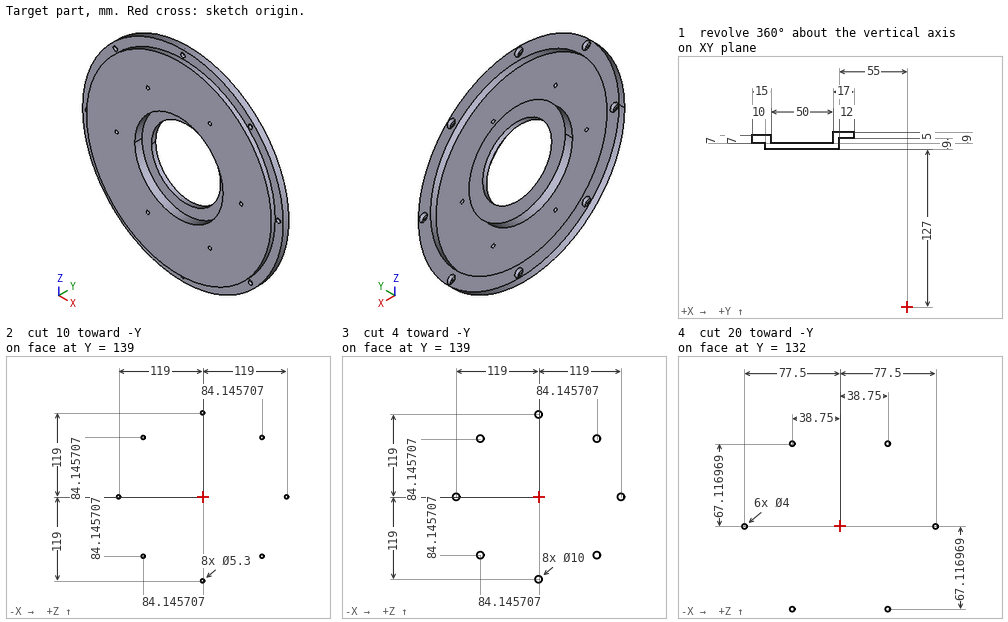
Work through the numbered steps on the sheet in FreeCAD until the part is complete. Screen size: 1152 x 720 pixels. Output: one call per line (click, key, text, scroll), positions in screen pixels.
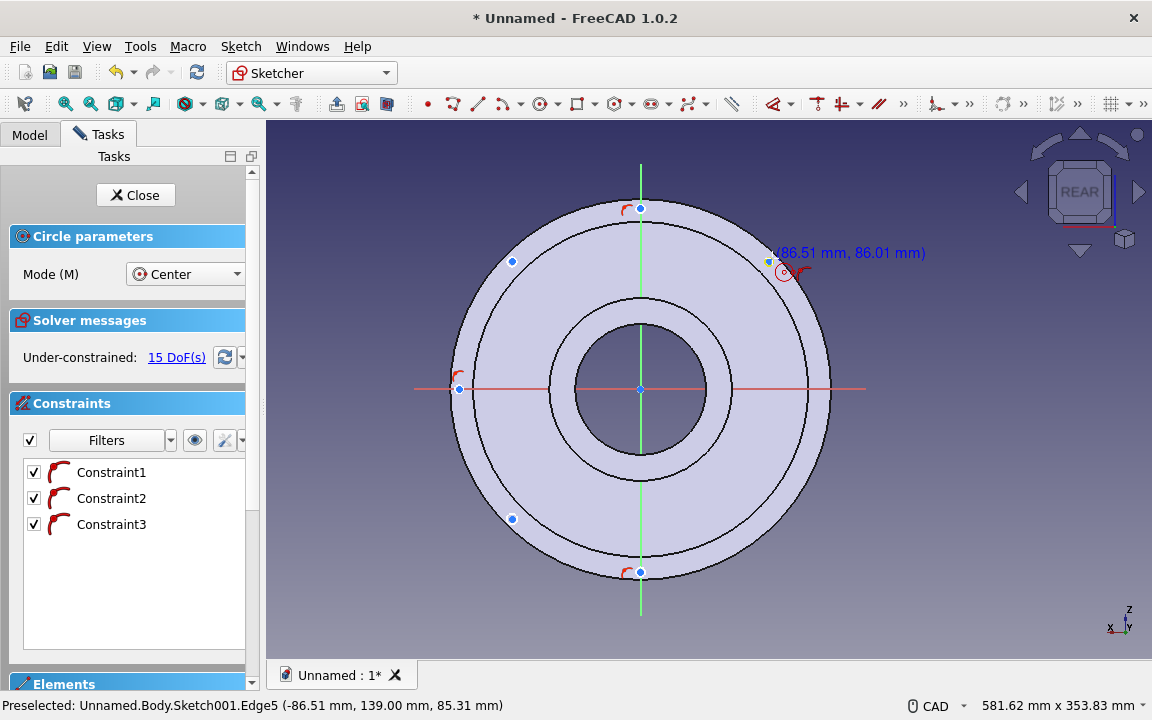
scroll(822, 389, up, 9)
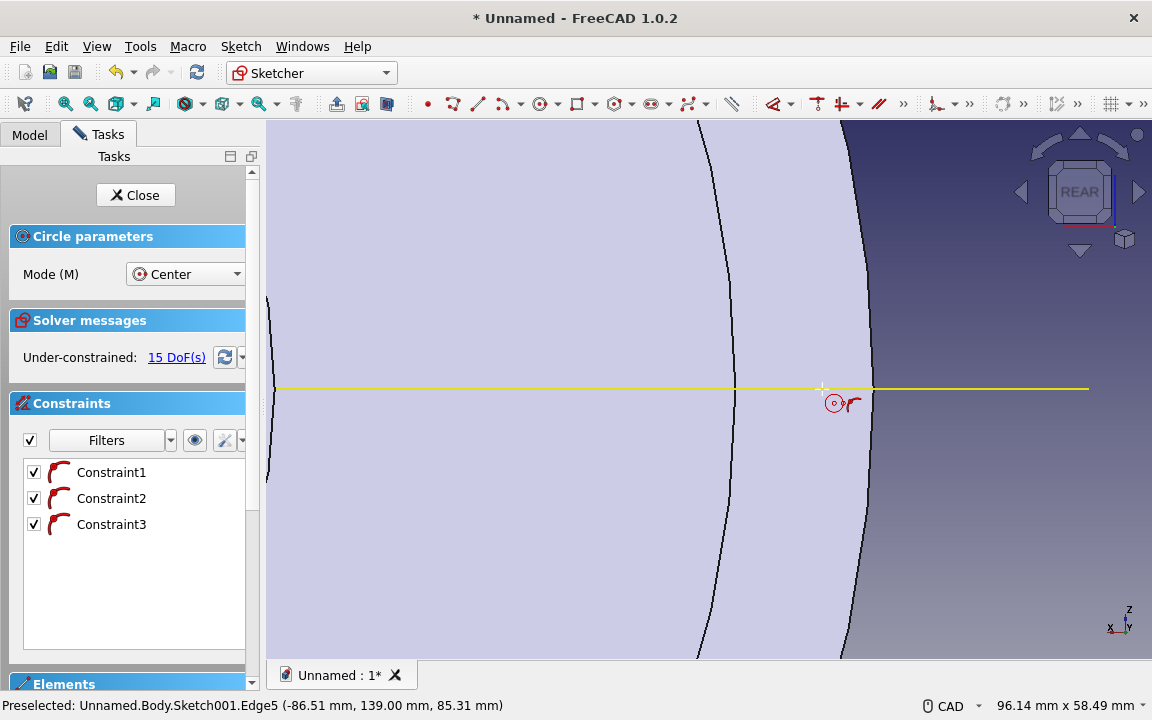
scroll(822, 390, down, 9)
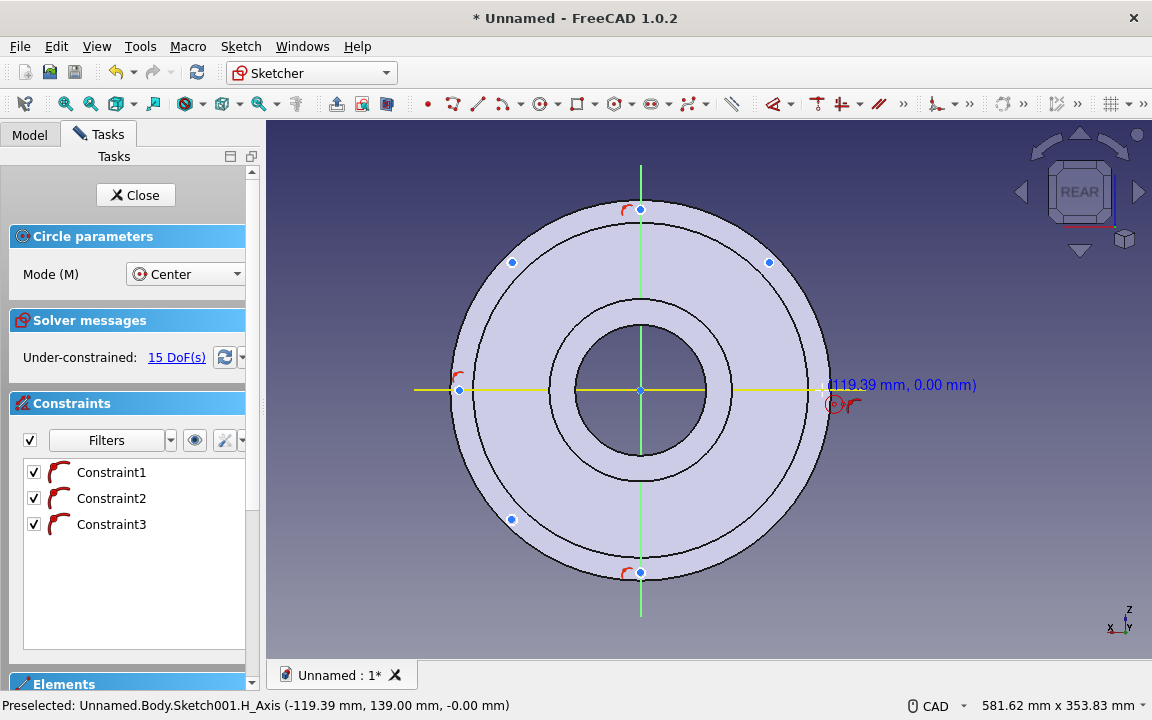
click(822, 390)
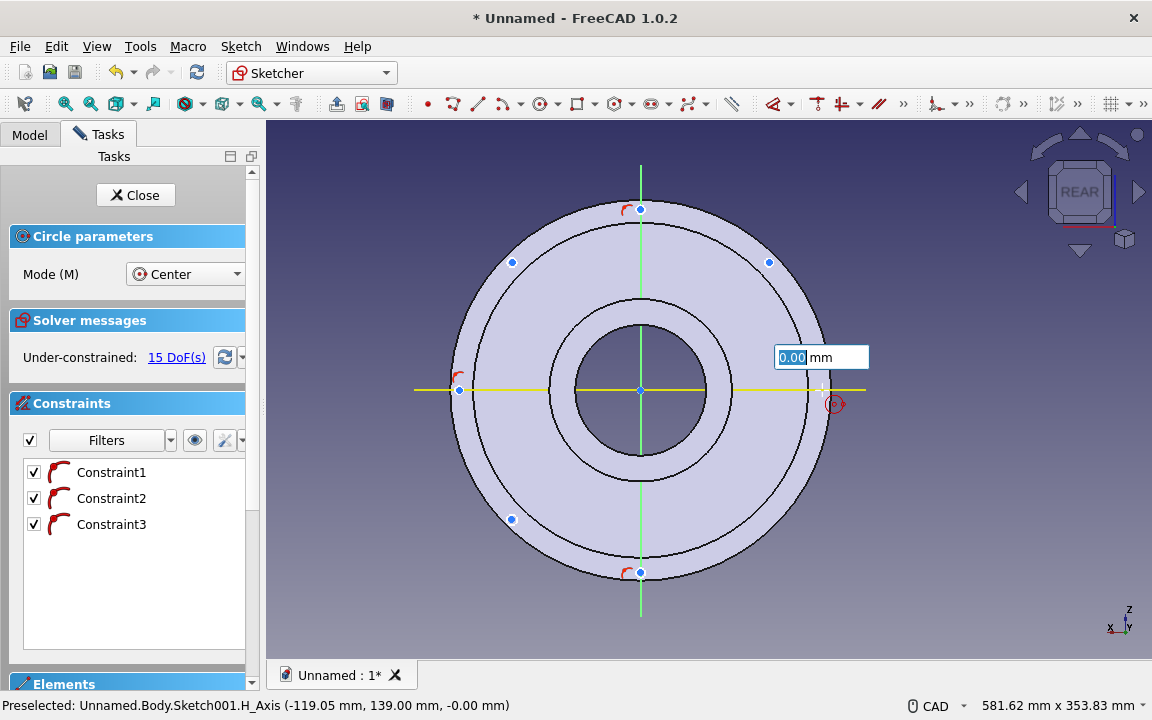
scroll(821, 394, up, 8)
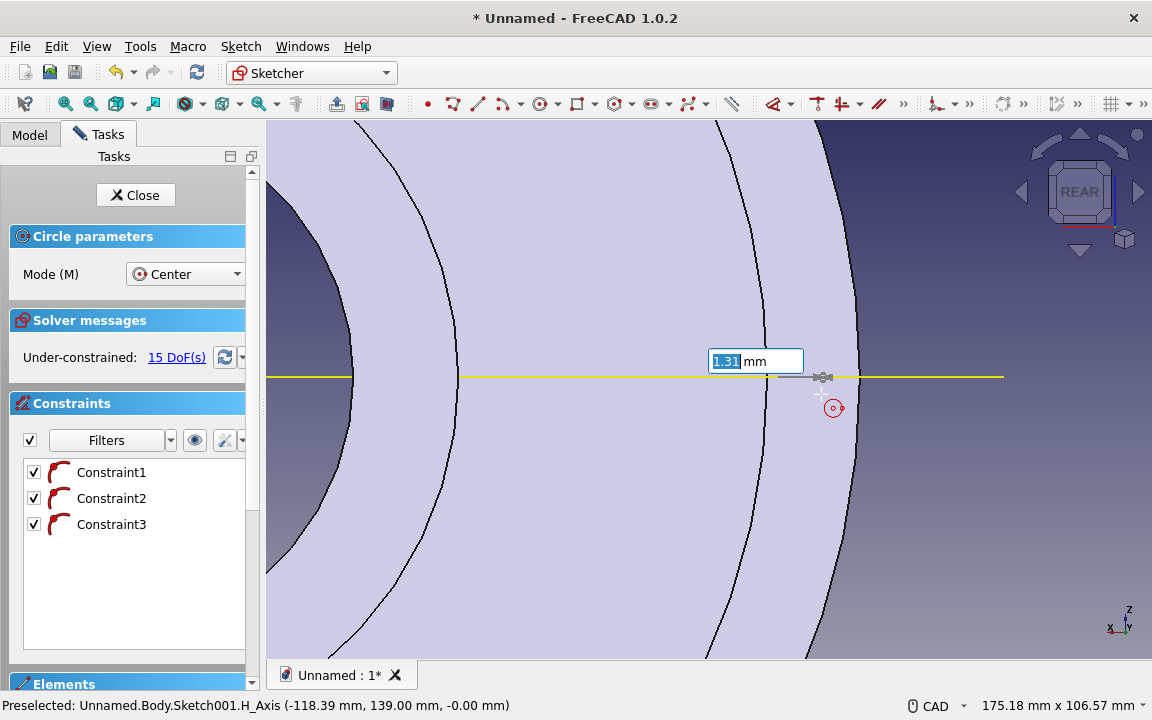
click(816, 392)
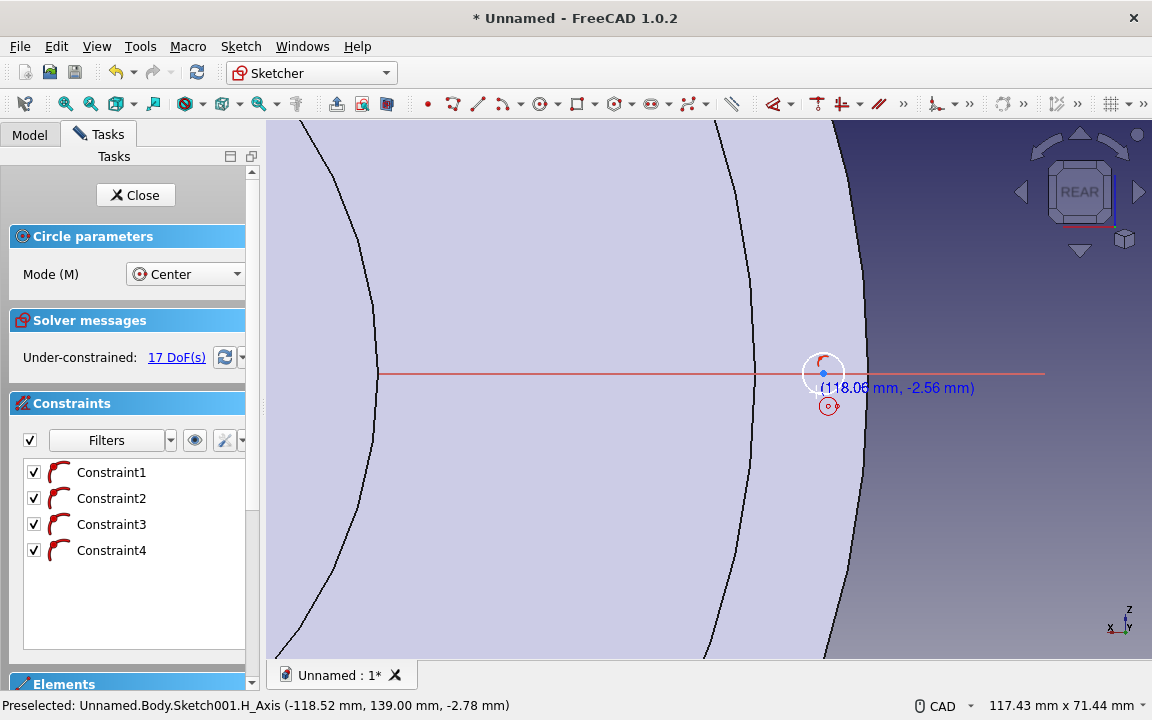
scroll(821, 394, down, 8)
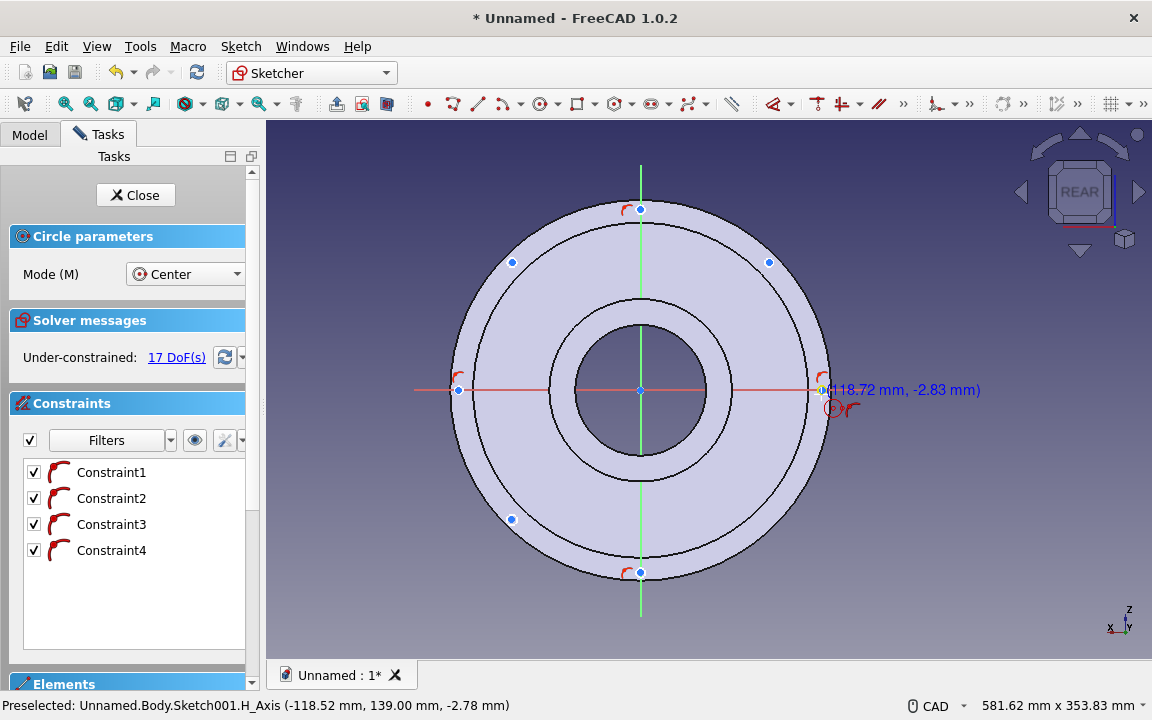
scroll(769, 518, up, 9)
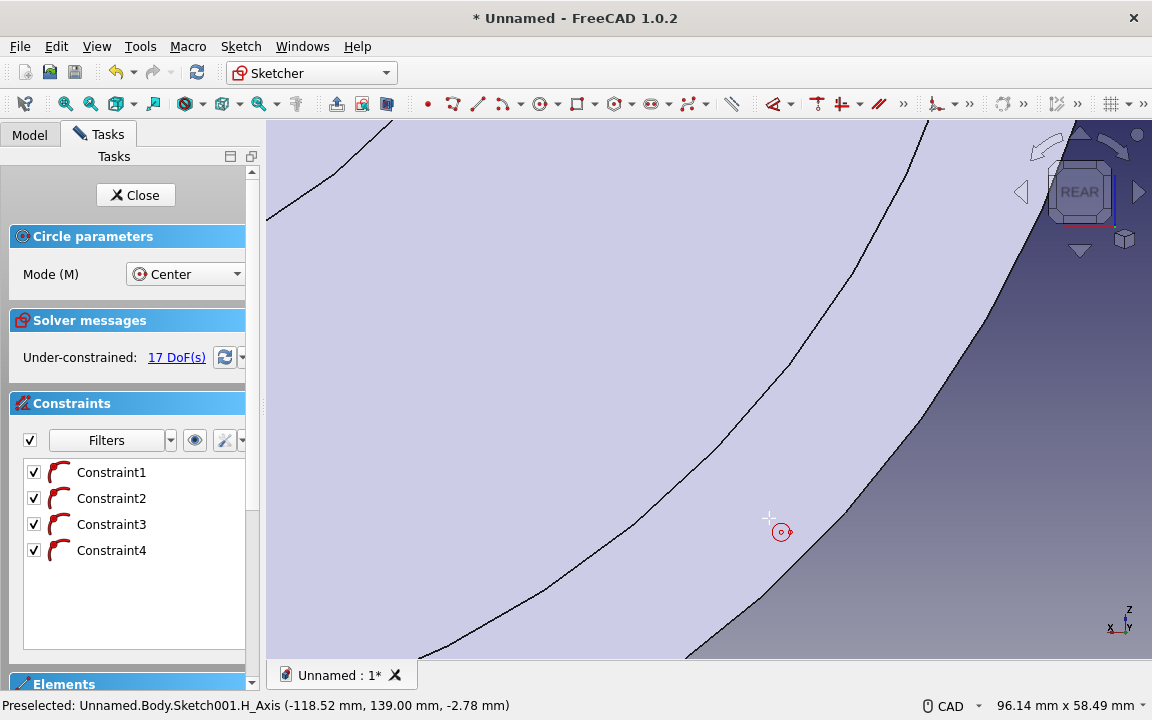
scroll(769, 518, down, 9)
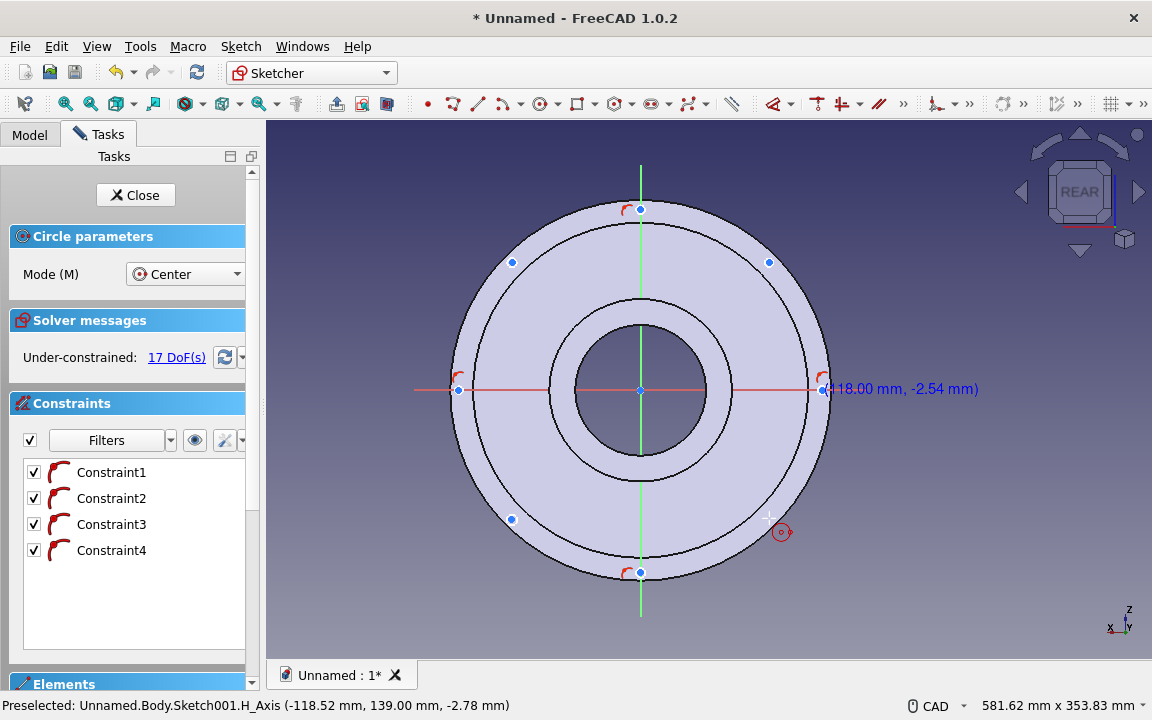
click(769, 518)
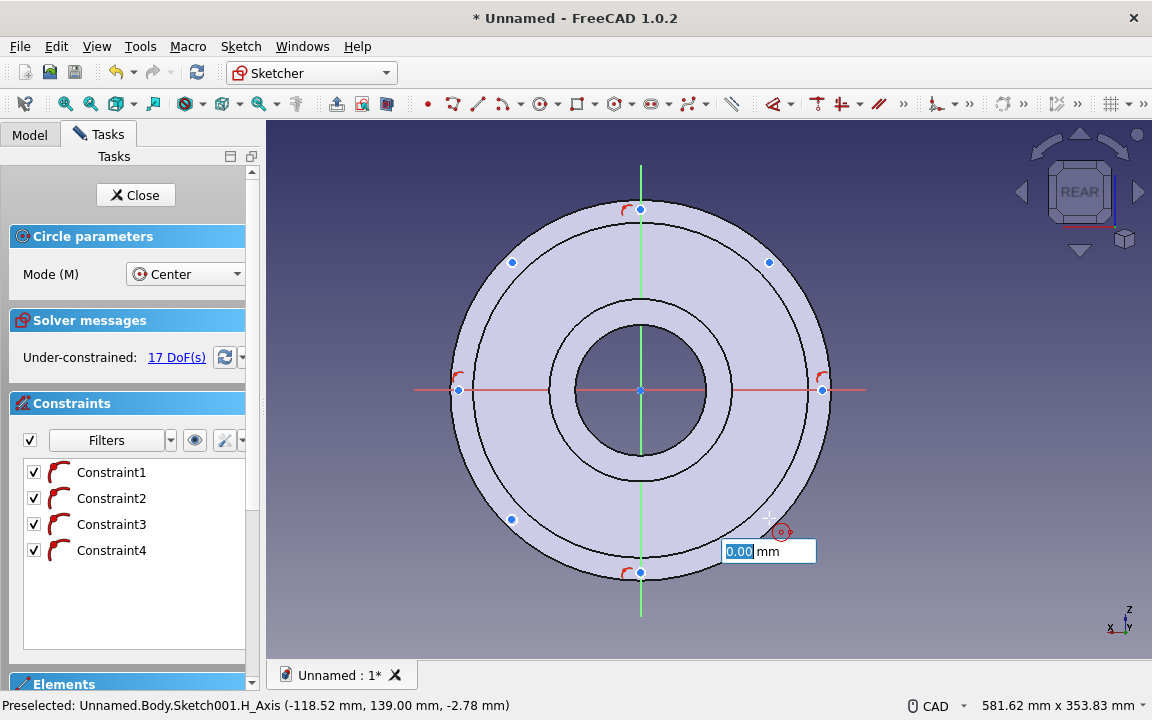
scroll(772, 516, up, 7)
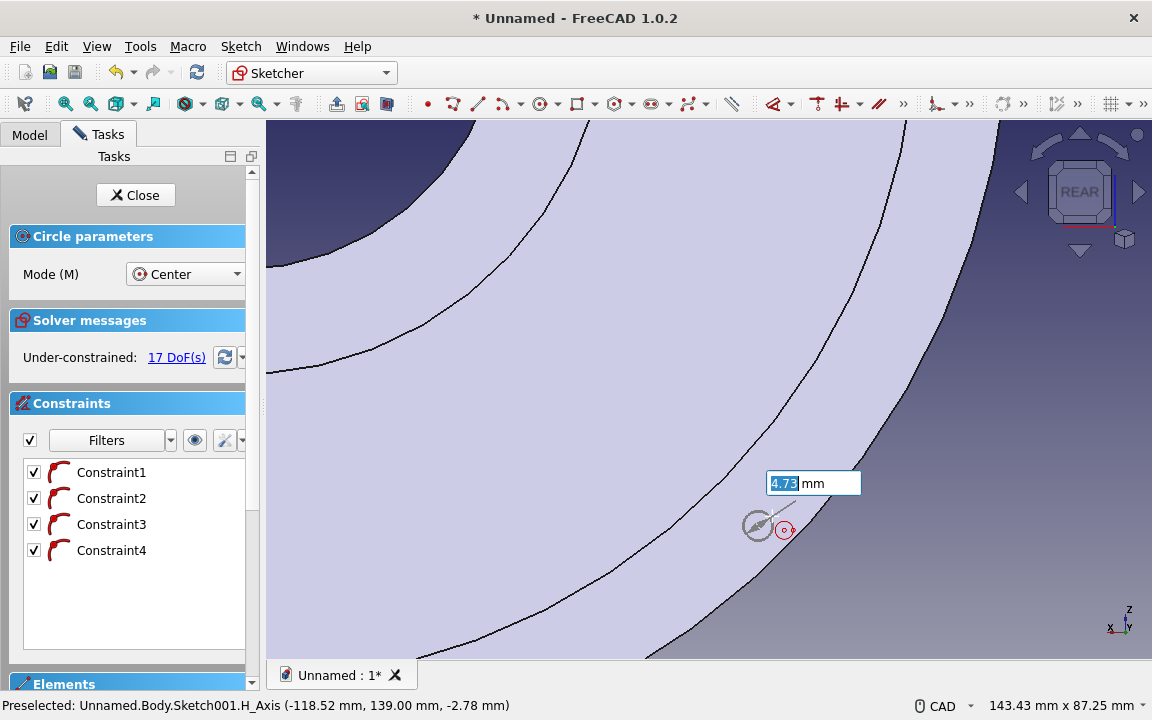
click(769, 512)
key(Escape)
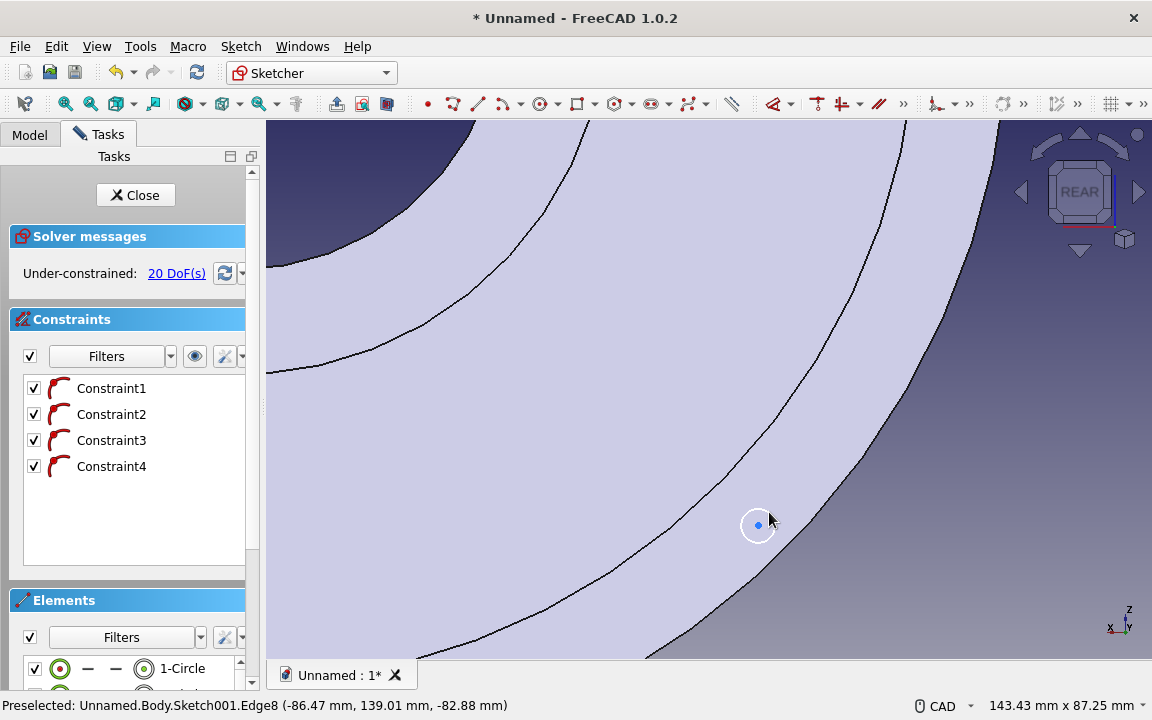
scroll(772, 516, down, 7)